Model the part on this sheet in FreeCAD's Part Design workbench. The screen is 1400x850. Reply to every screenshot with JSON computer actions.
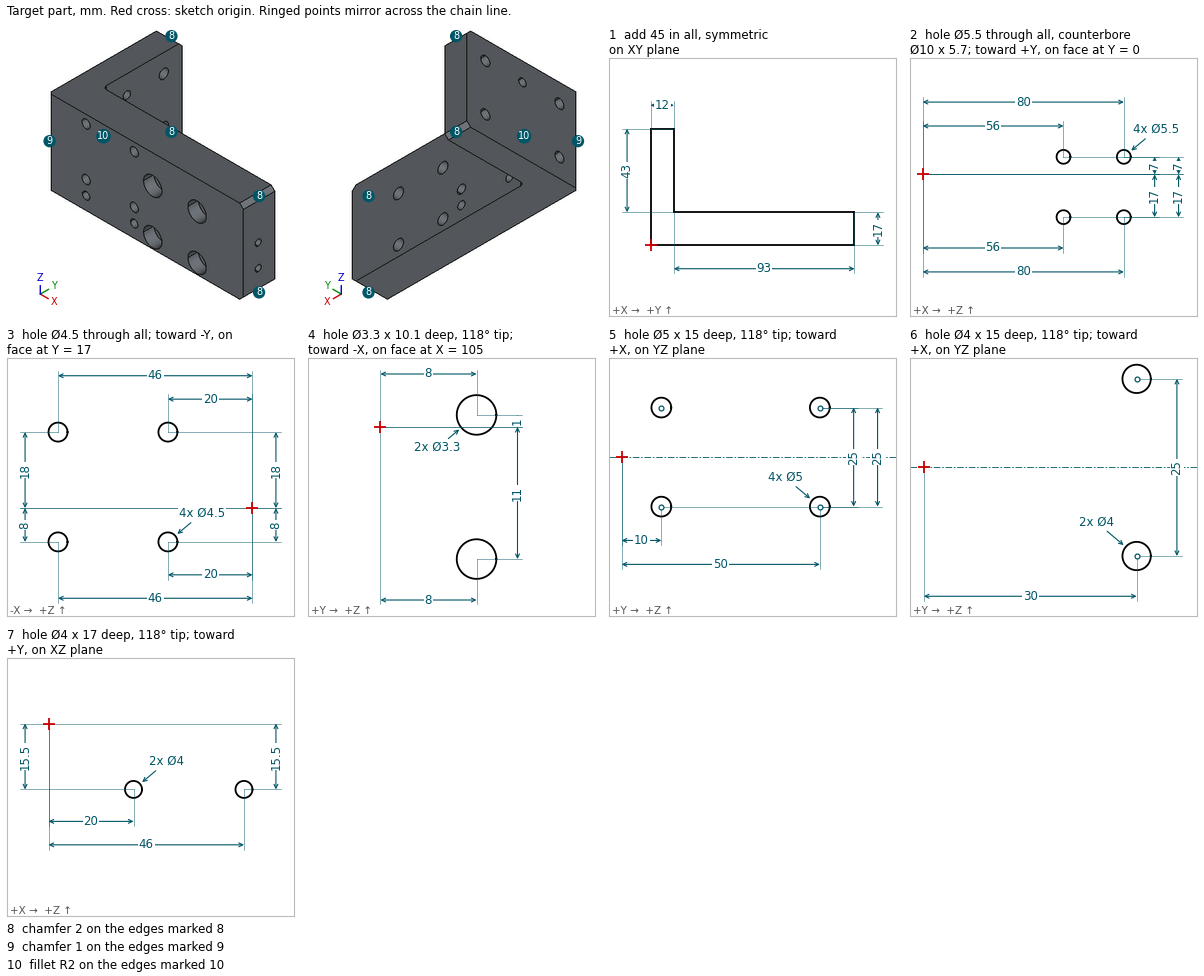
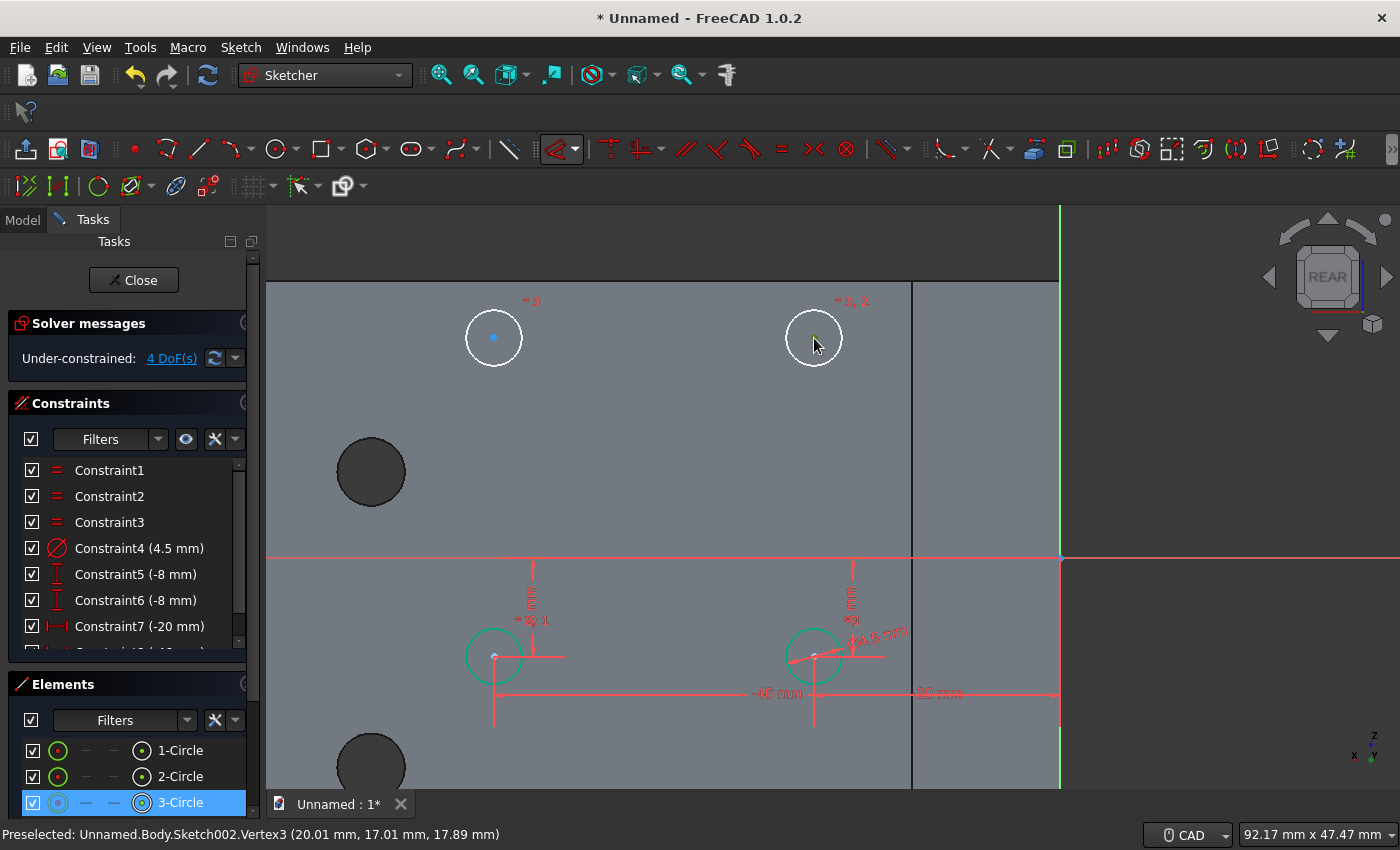
{"action": "left_click", "coordinate": [578, 150]}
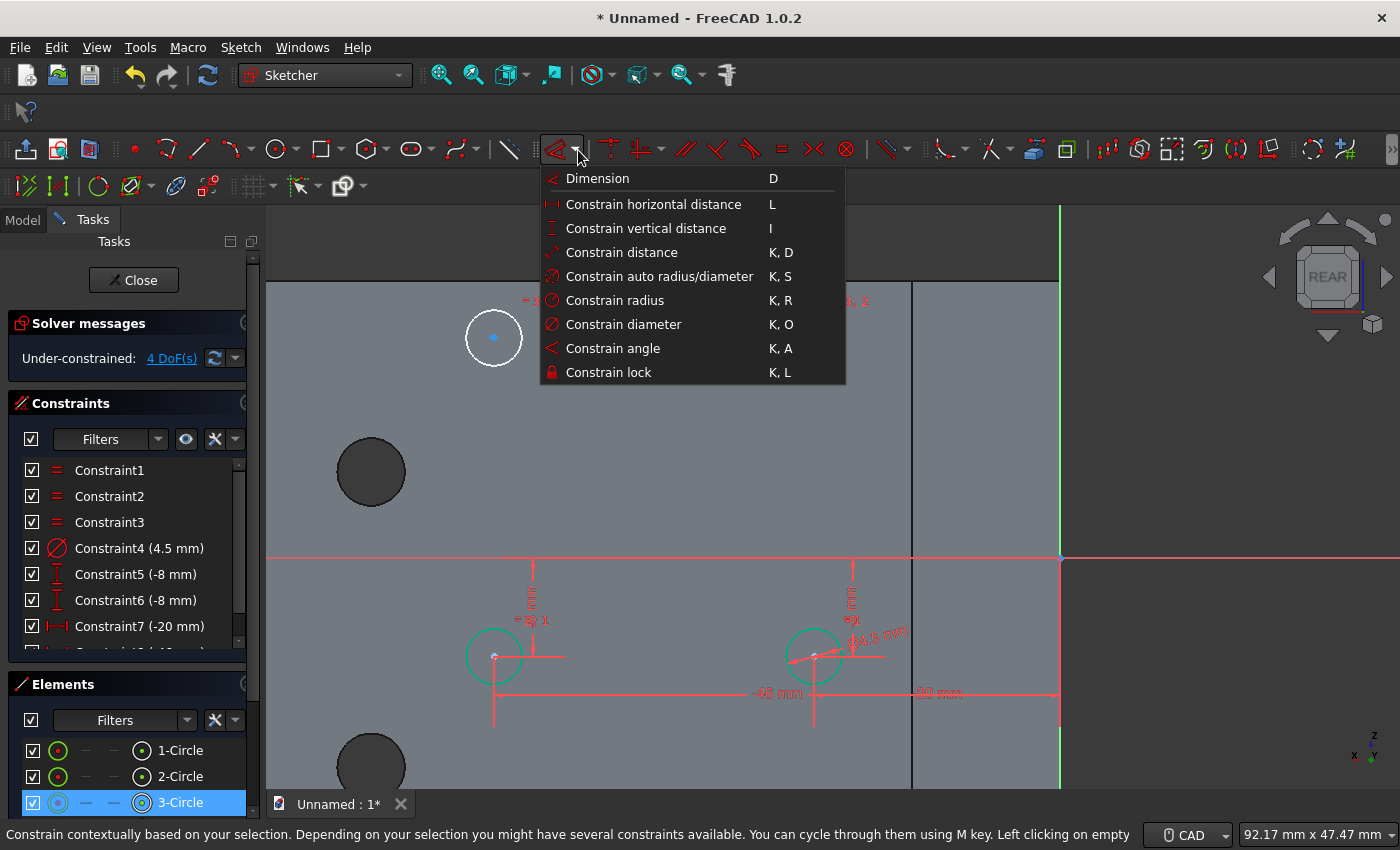
{"action": "left_click", "coordinate": [693, 204]}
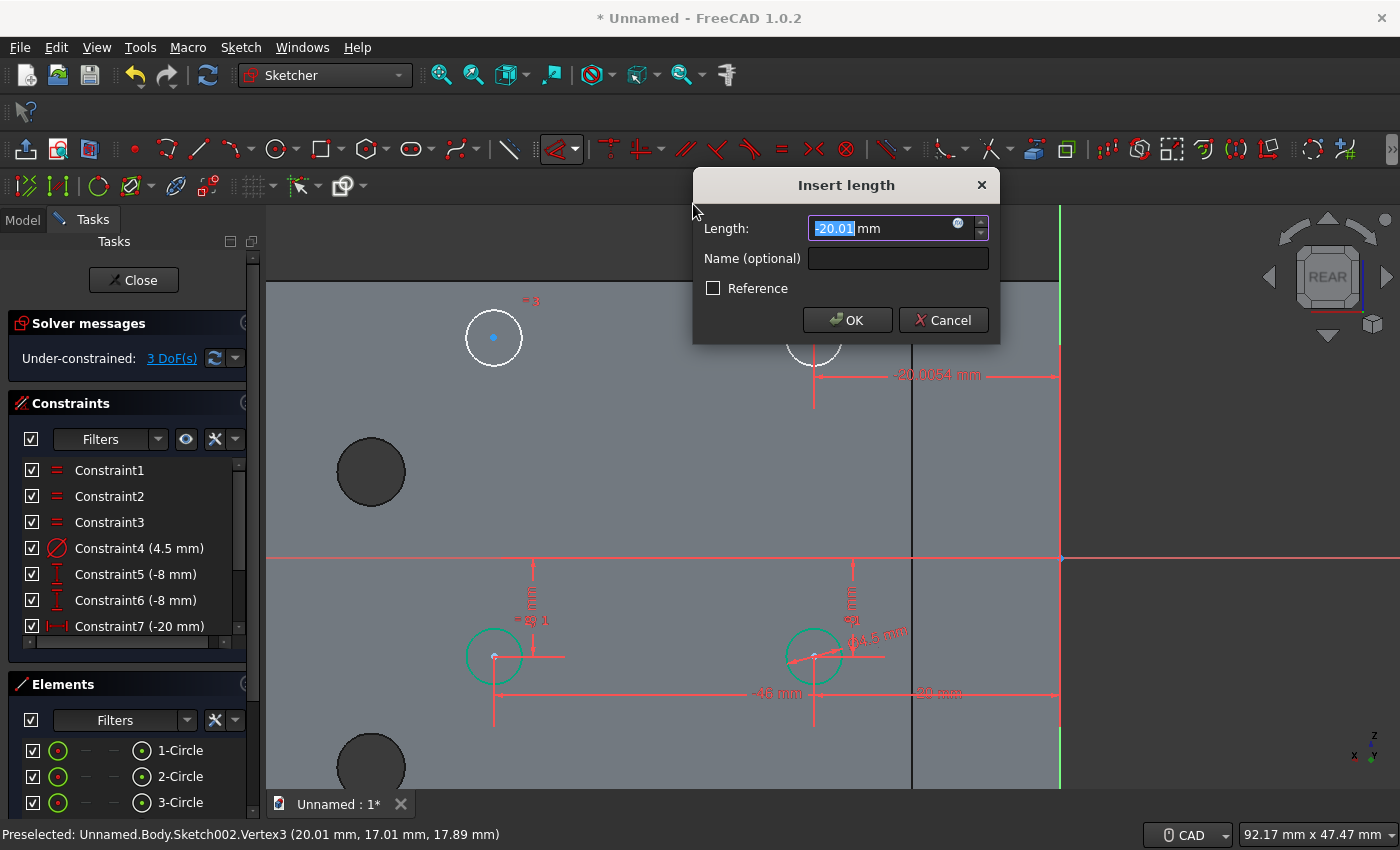
{"action": "type", "text": "-20"}
{"action": "key", "text": "Return"}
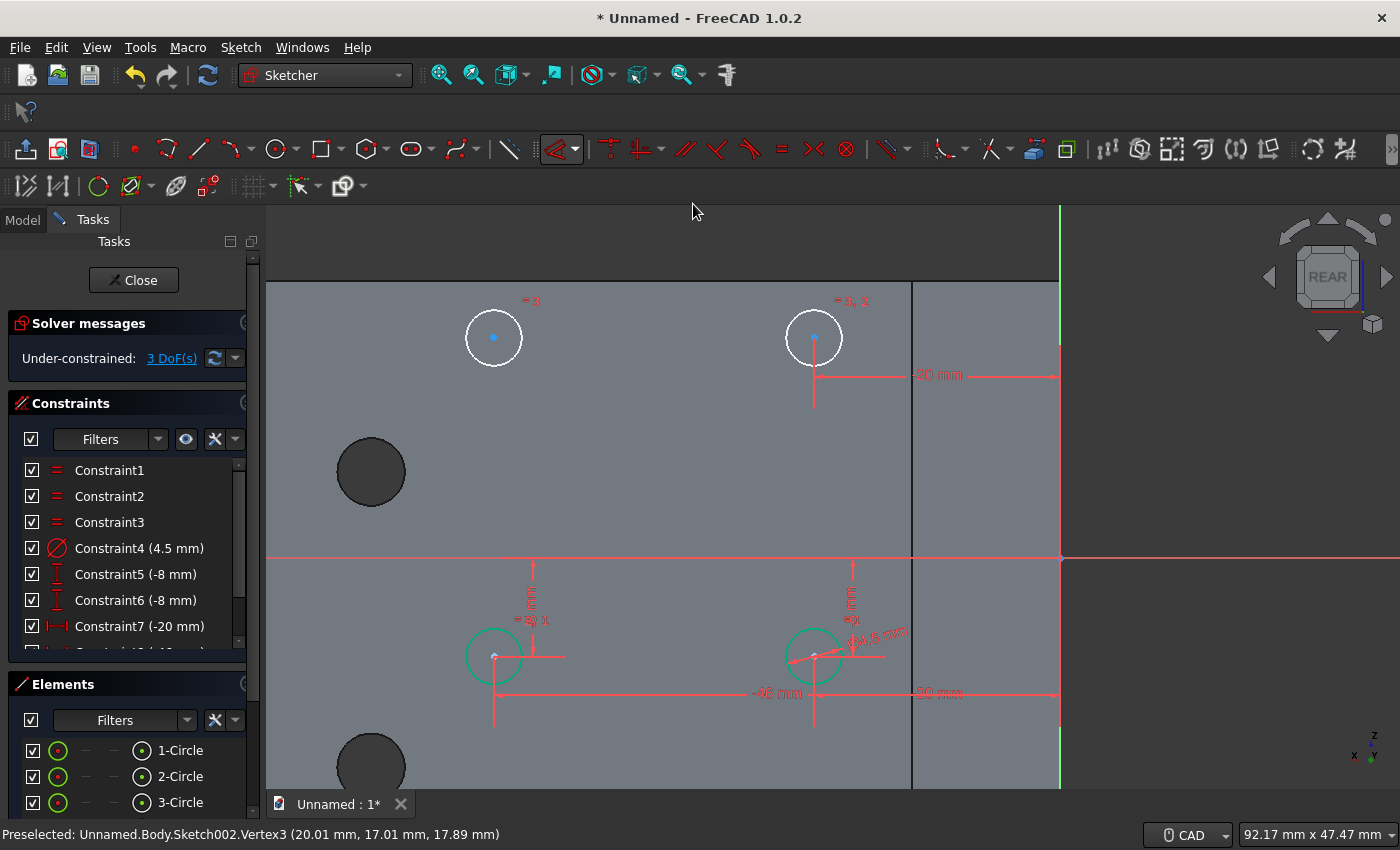
{"action": "left_click", "coordinate": [814, 338]}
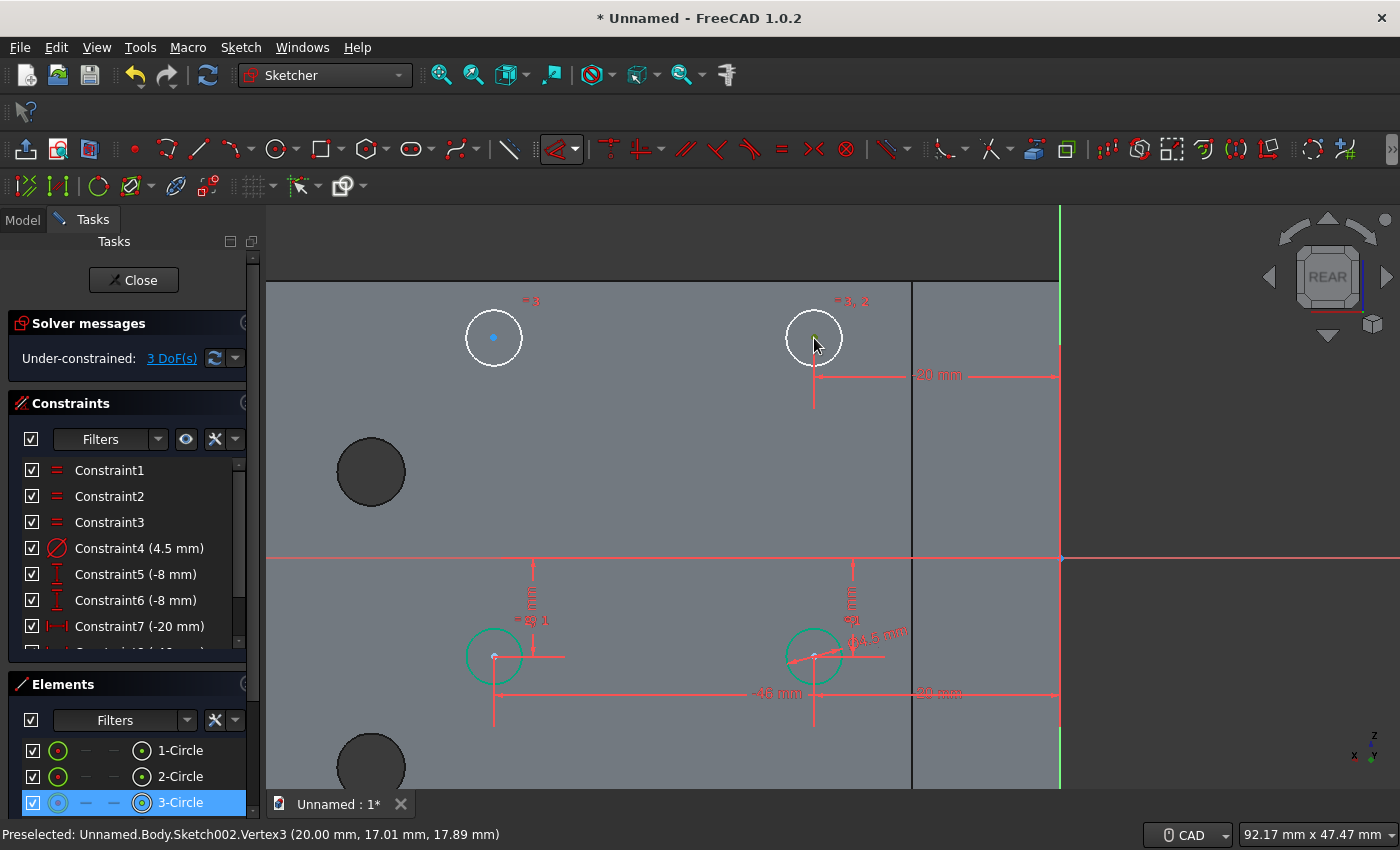
{"action": "left_click", "coordinate": [578, 150]}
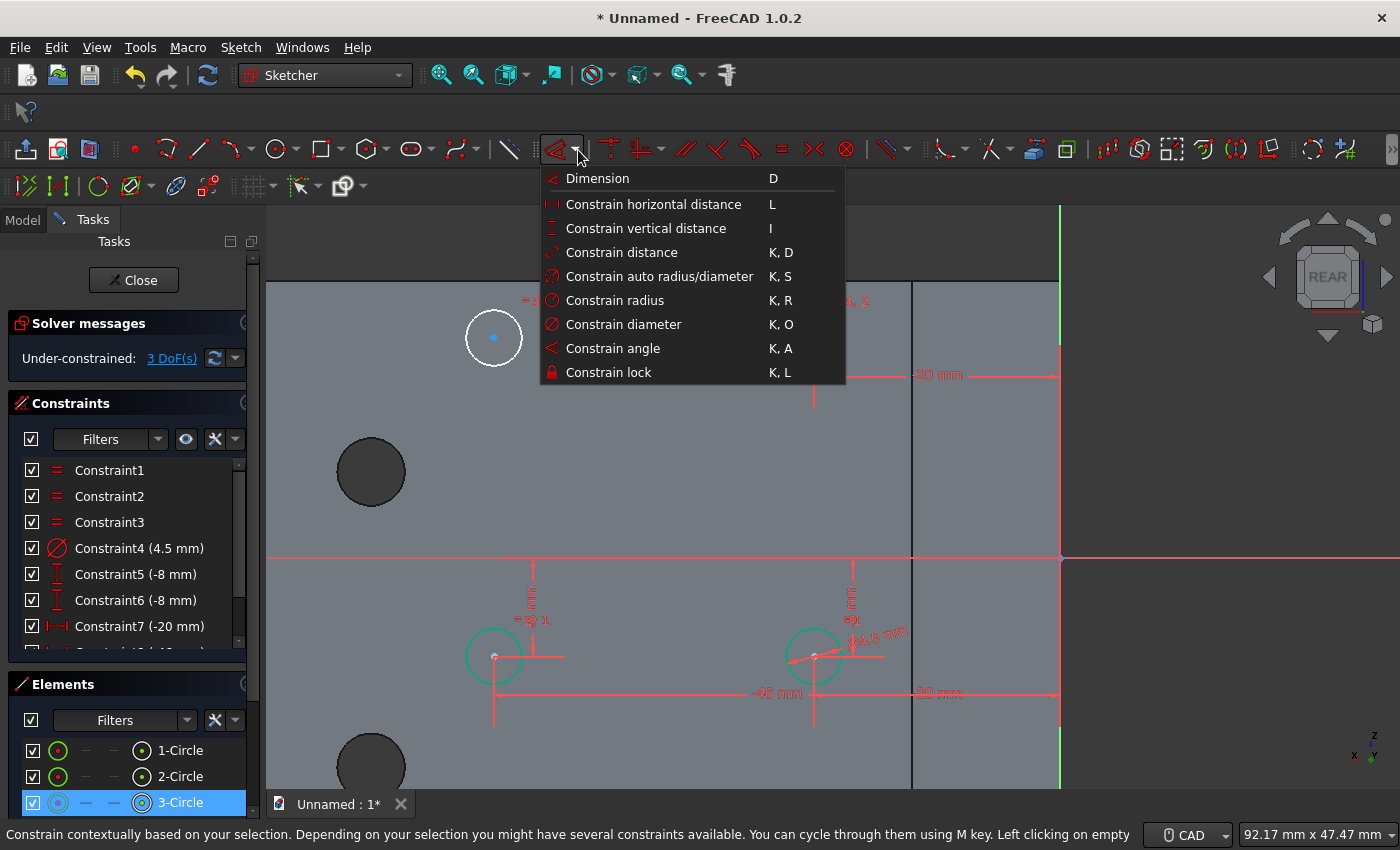
{"action": "left_click", "coordinate": [693, 228]}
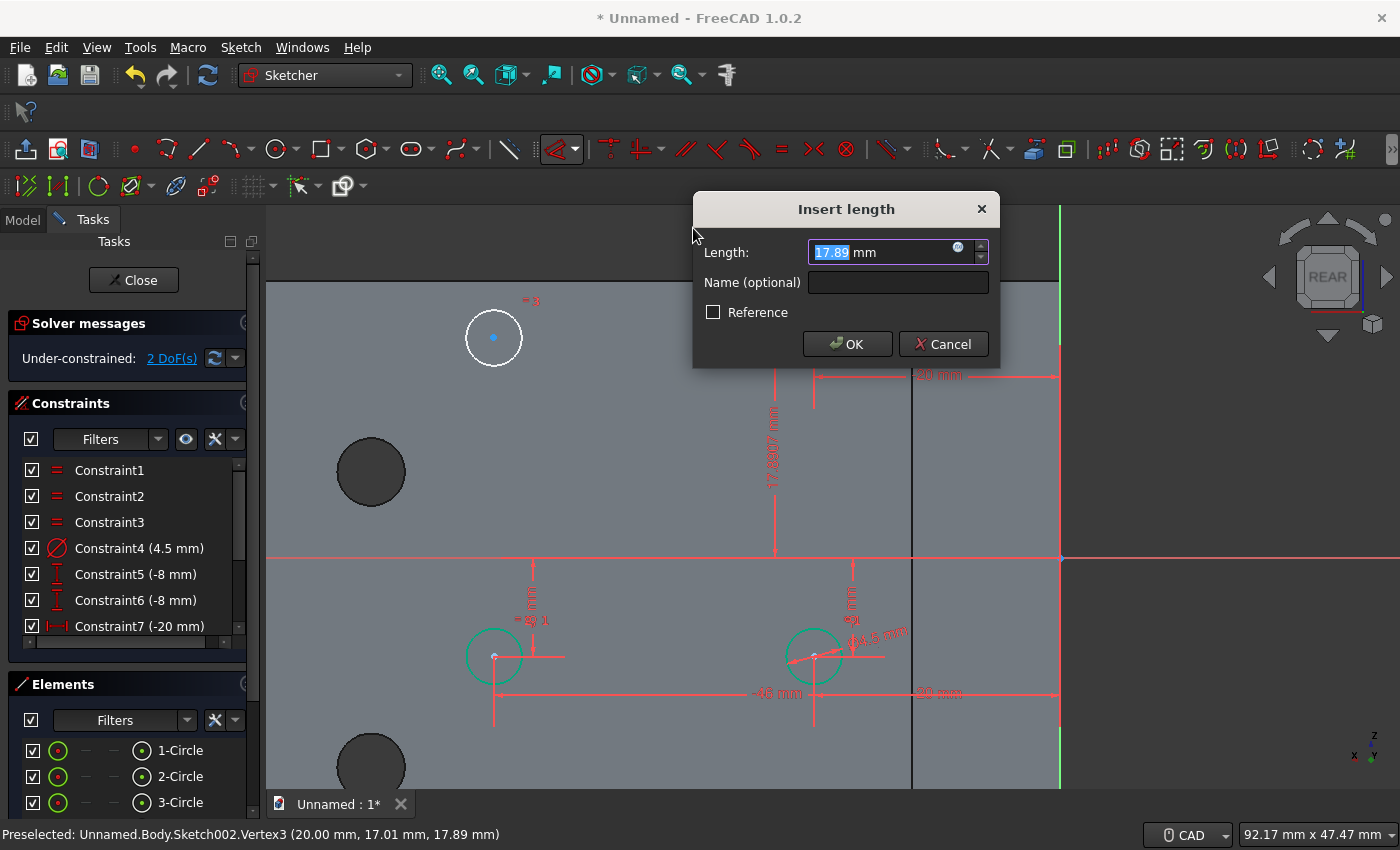
{"action": "type", "text": "18"}
{"action": "key", "text": "Return"}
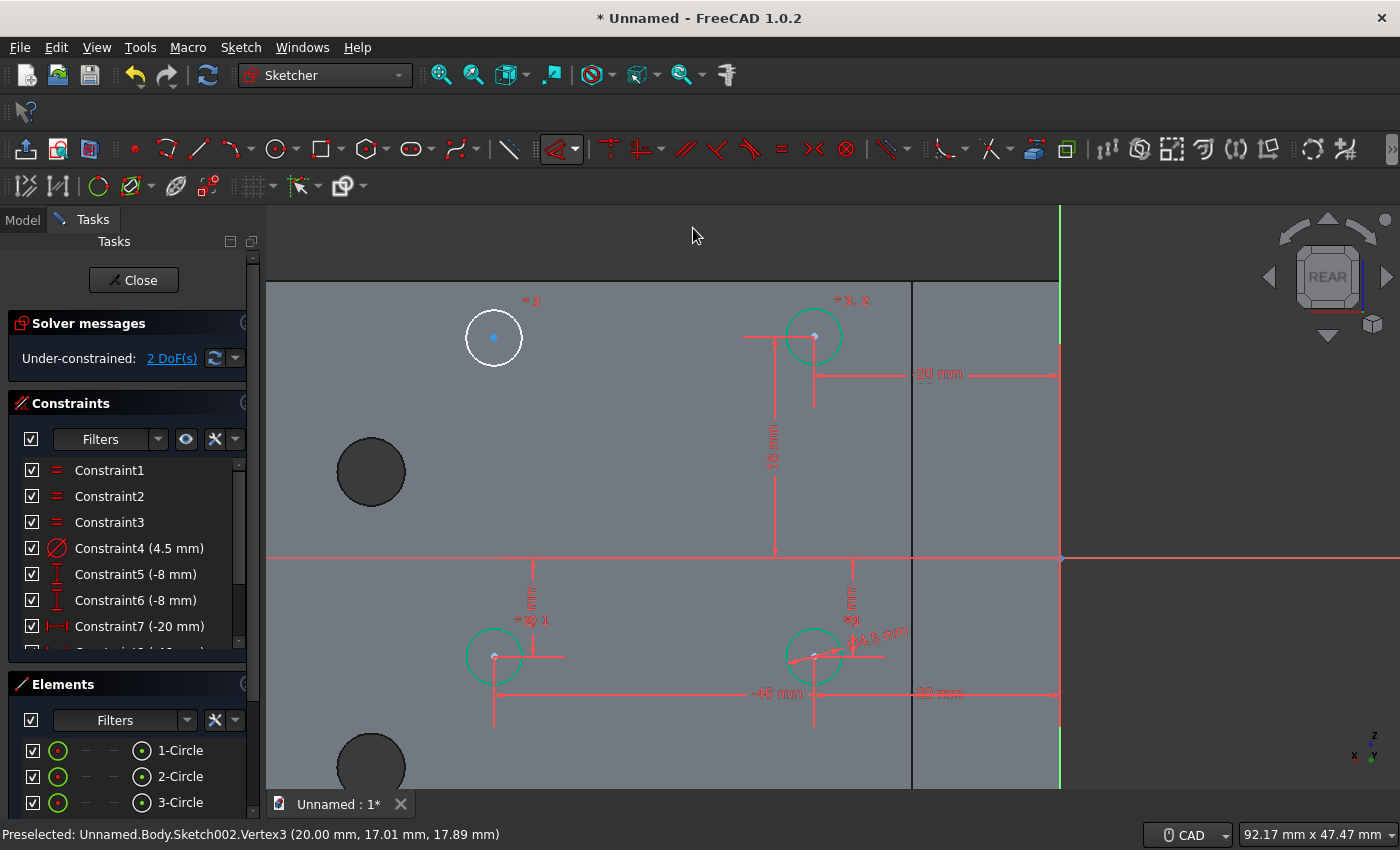
{"action": "left_click", "coordinate": [494, 338]}